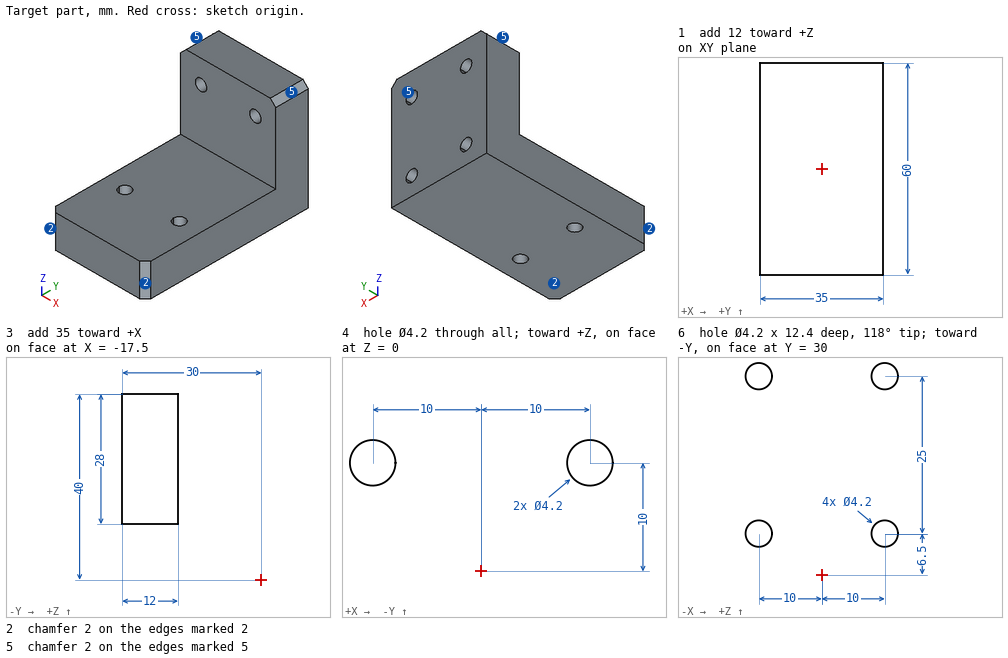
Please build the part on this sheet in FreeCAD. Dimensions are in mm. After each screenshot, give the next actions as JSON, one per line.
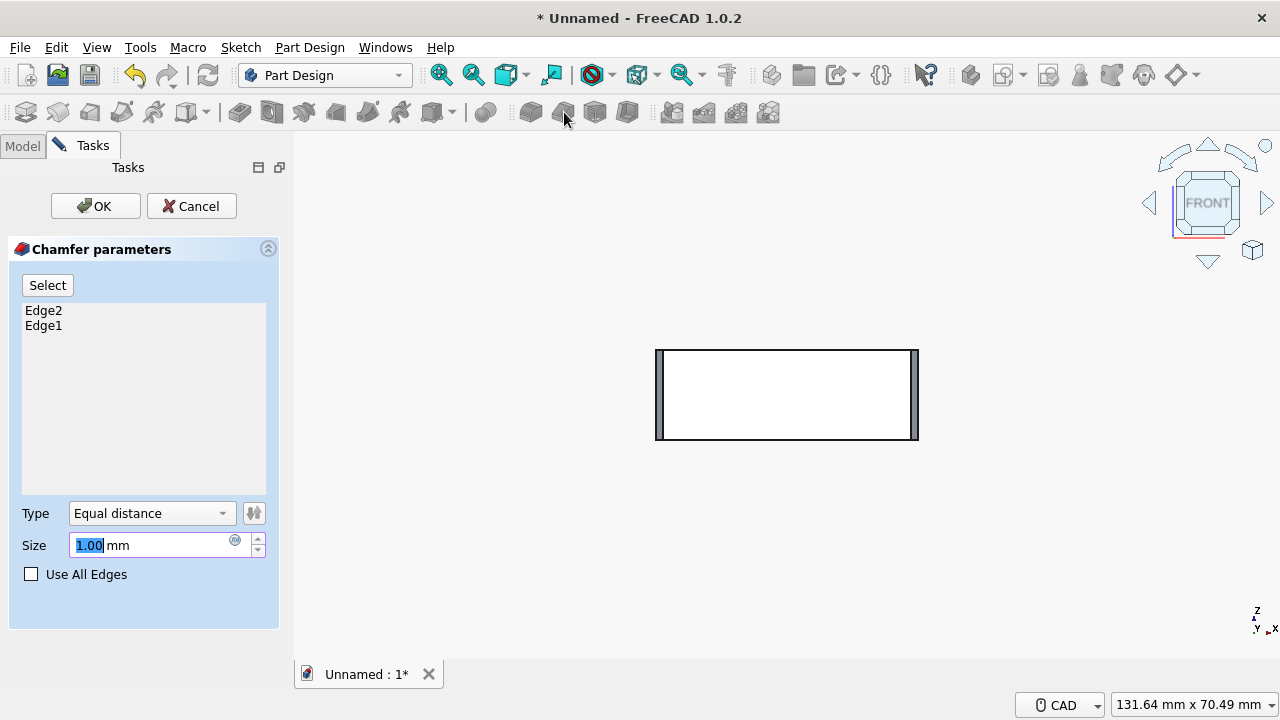
{"action": "type", "text": "2"}
{"action": "key", "text": "Tab"}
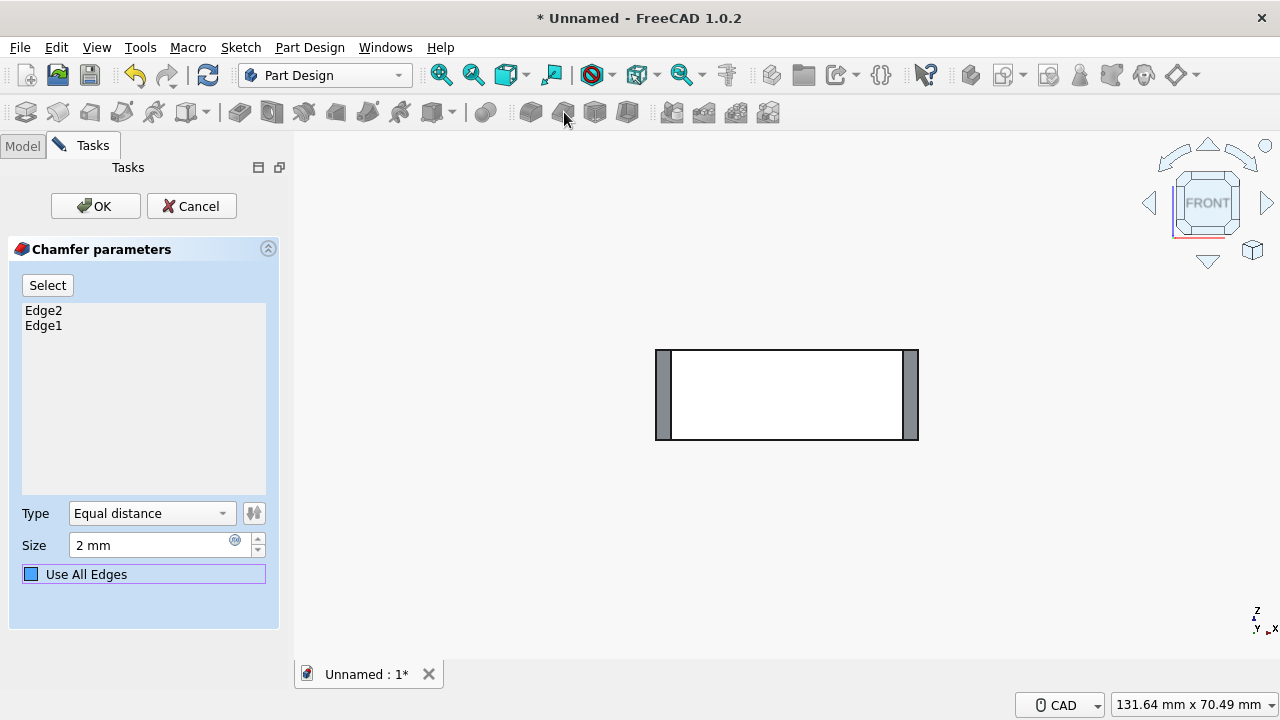
{"action": "left_click", "coordinate": [96, 206]}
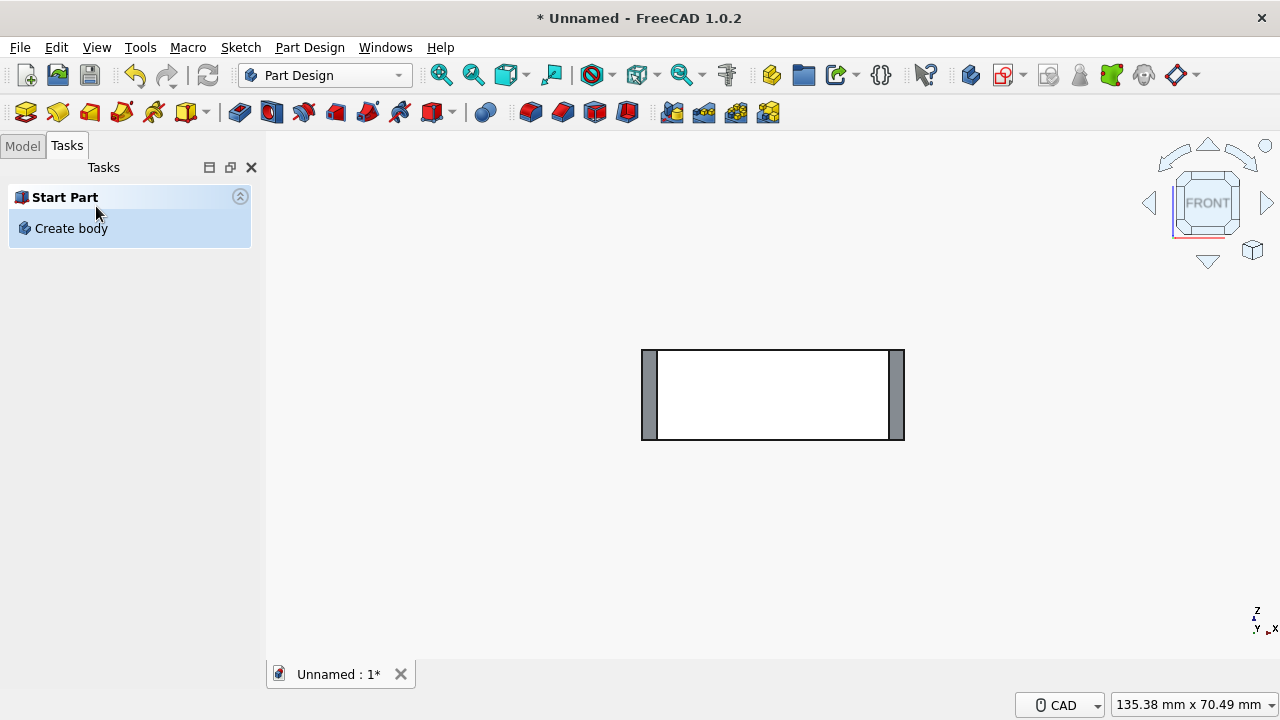
{"action": "left_click", "coordinate": [442, 76]}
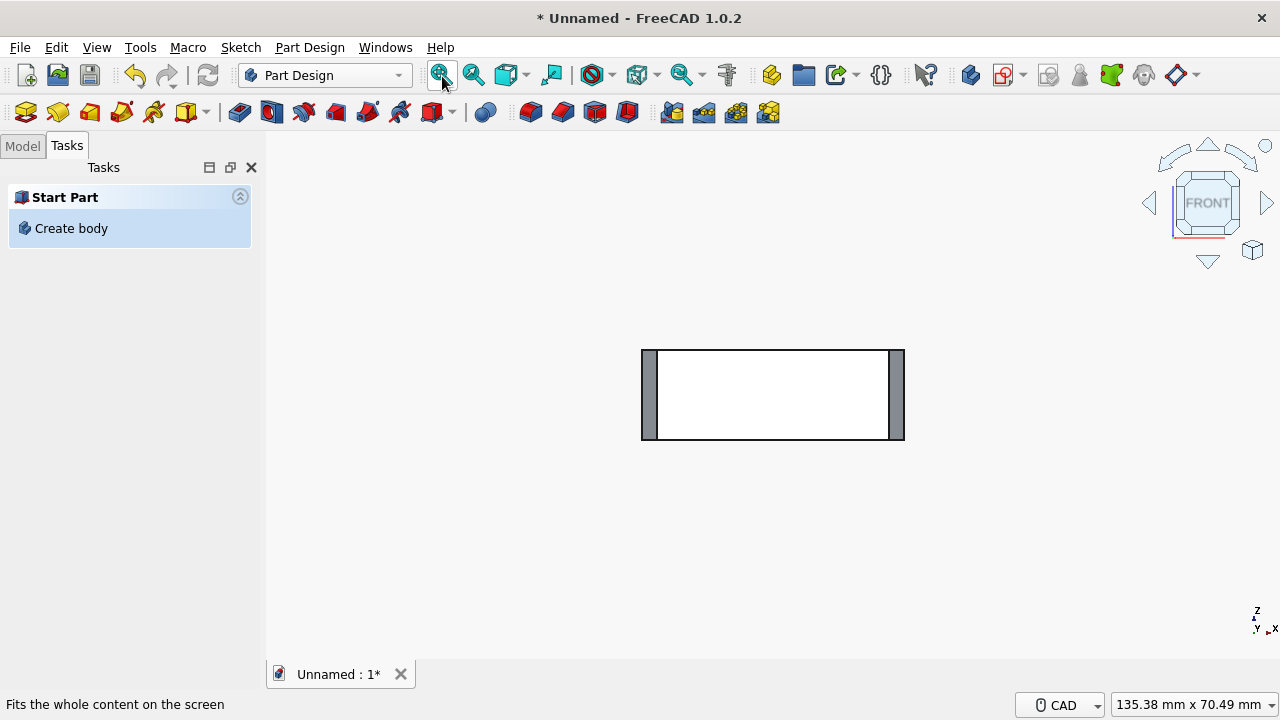
{"action": "key", "text": "6"}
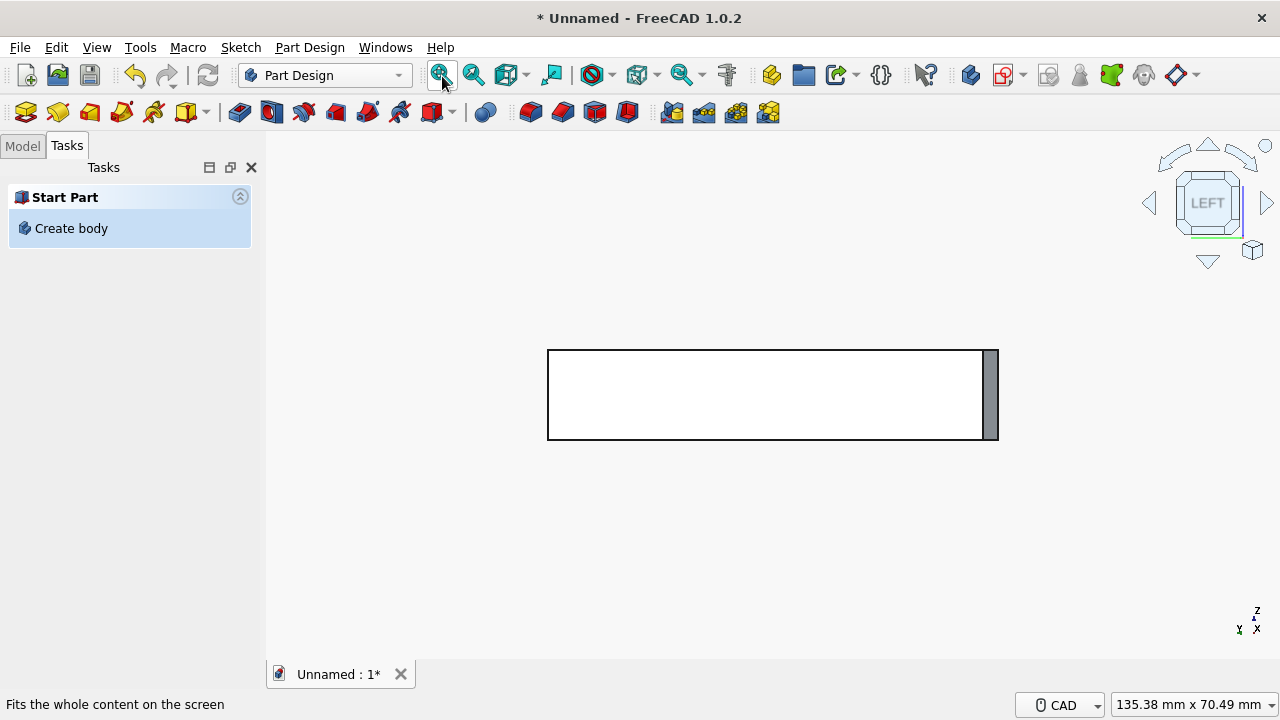
{"action": "left_click", "coordinate": [442, 76]}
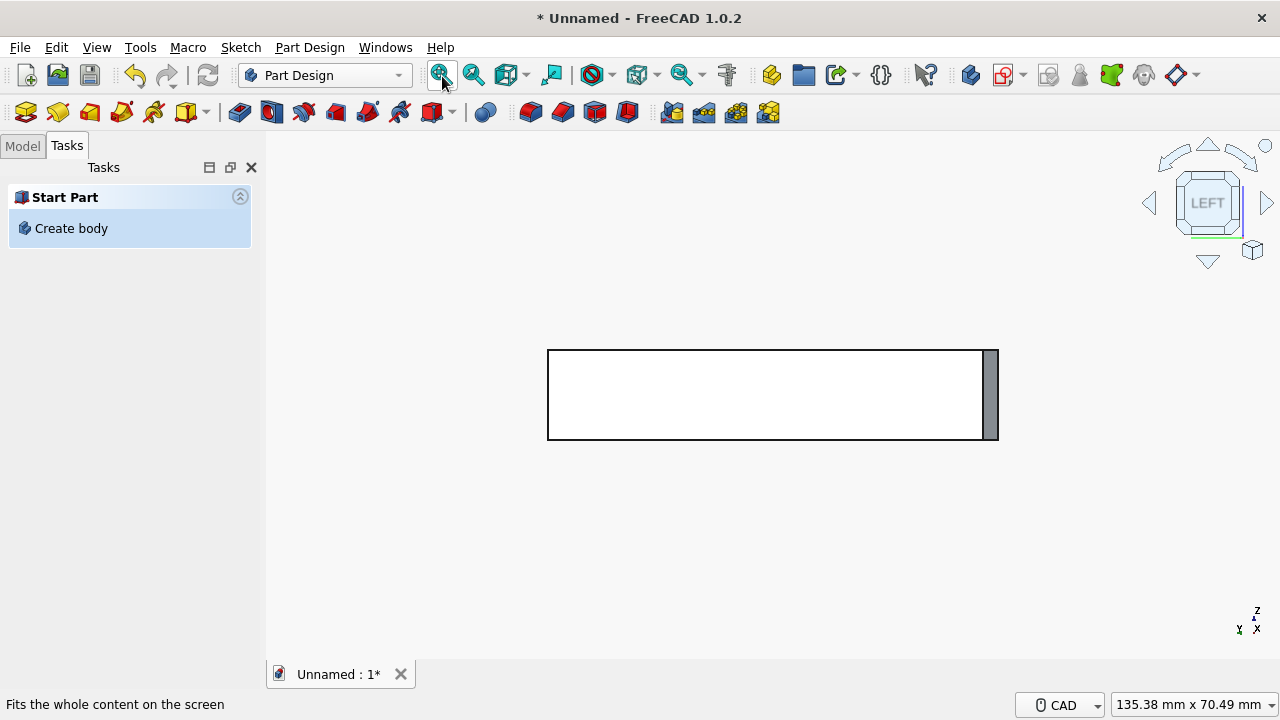
{"action": "left_click", "coordinate": [641, 394]}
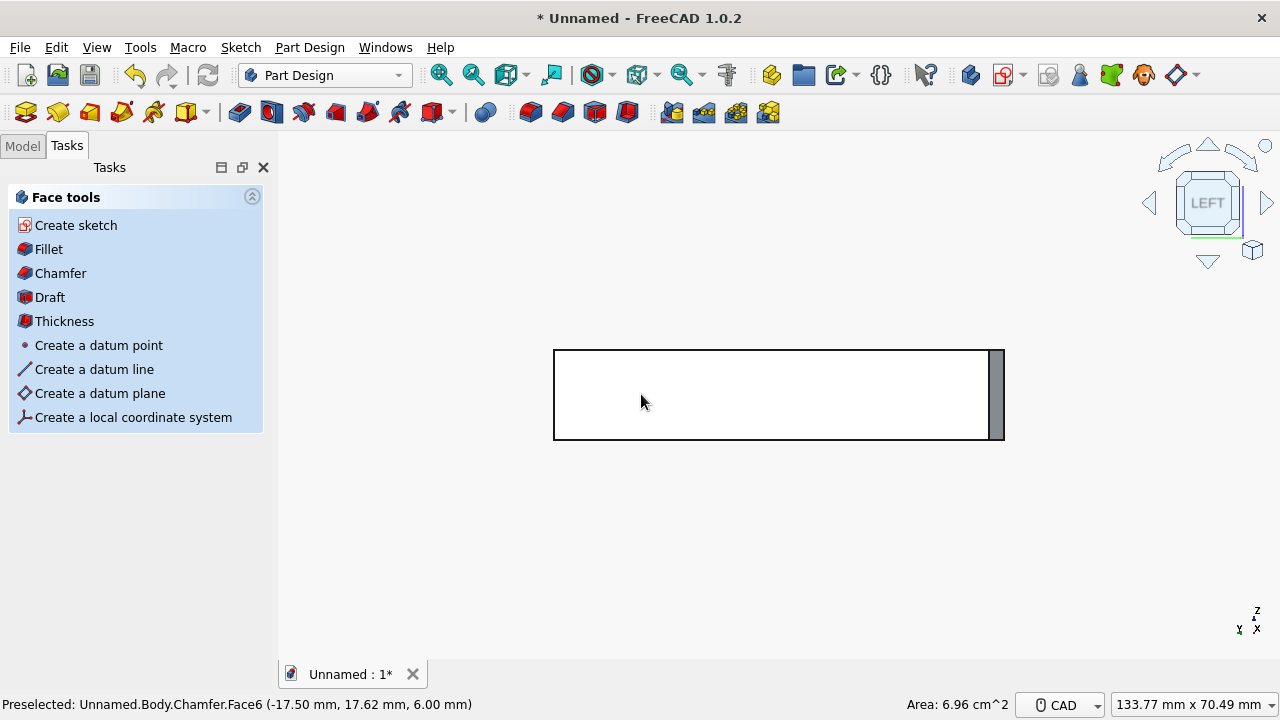
{"action": "left_click", "coordinate": [1004, 76]}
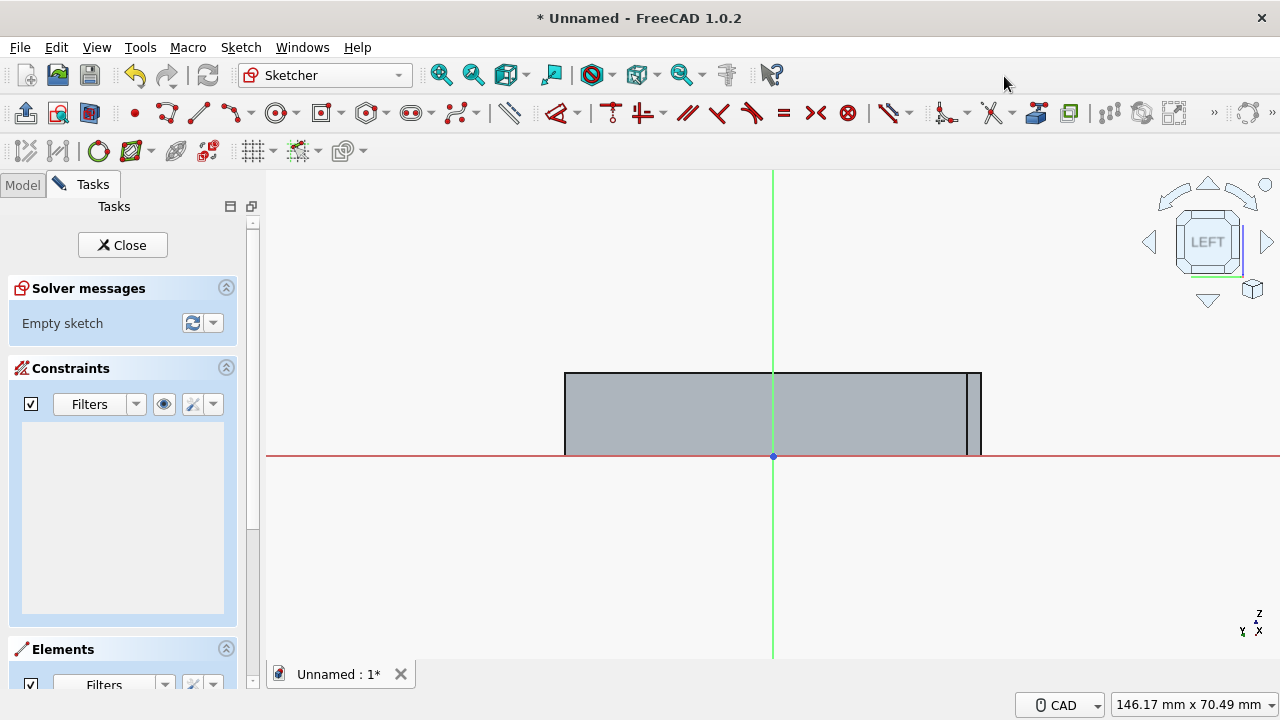
{"action": "scroll", "coordinate": [865, 631], "scroll_direction": "down", "scroll_amount": 1}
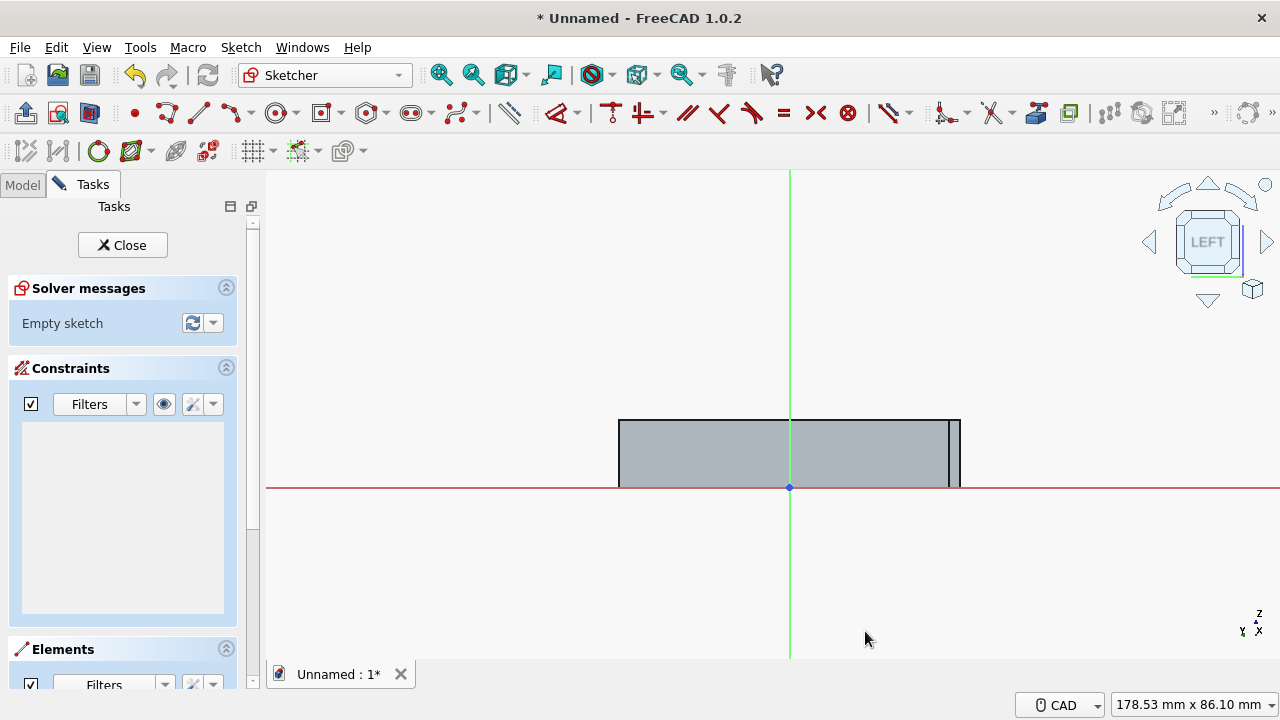
{"action": "left_click", "coordinate": [344, 114]}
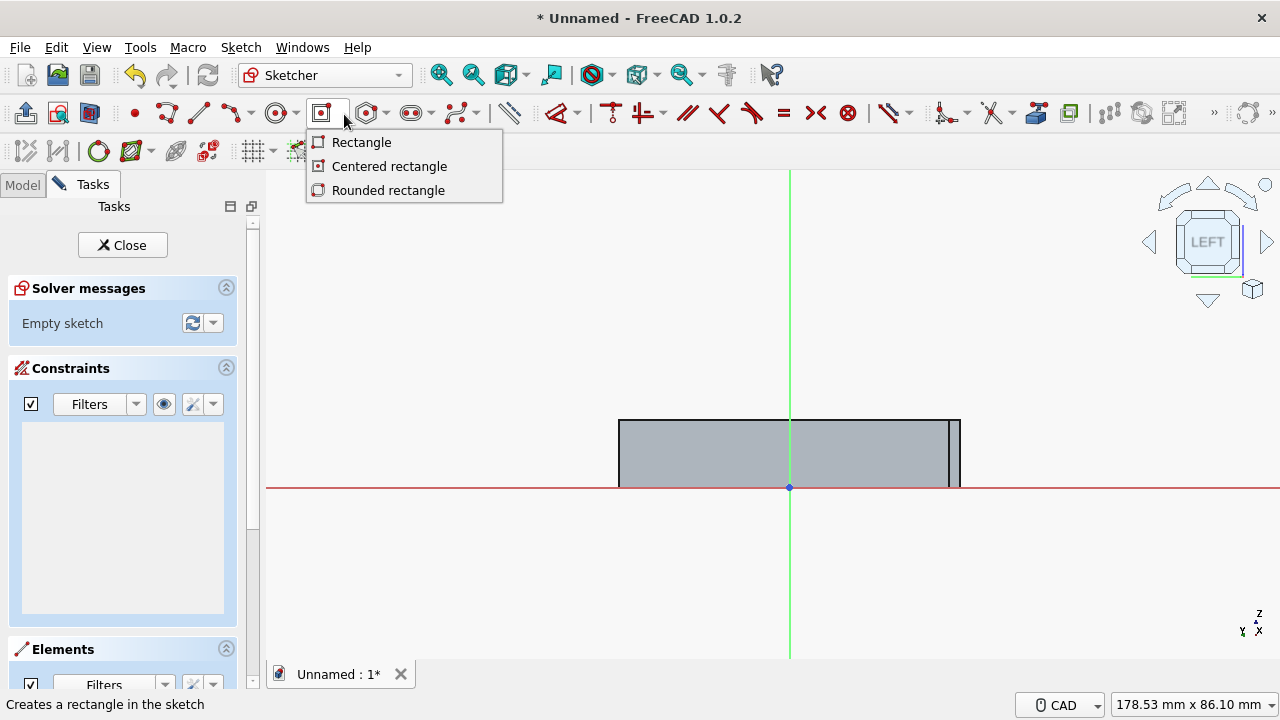
{"action": "left_click", "coordinate": [404, 142]}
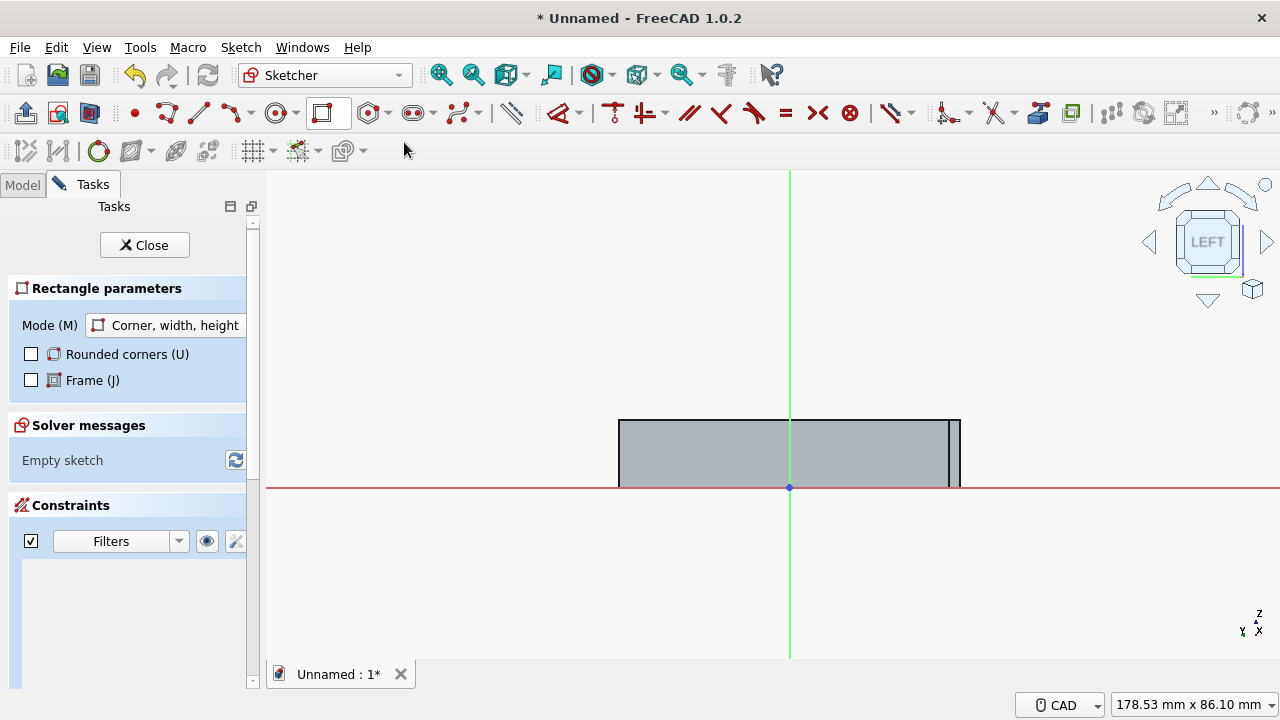
{"action": "left_click", "coordinate": [619, 261]}
{"action": "left_click", "coordinate": [688, 420]}
{"action": "key", "text": "Escape"}